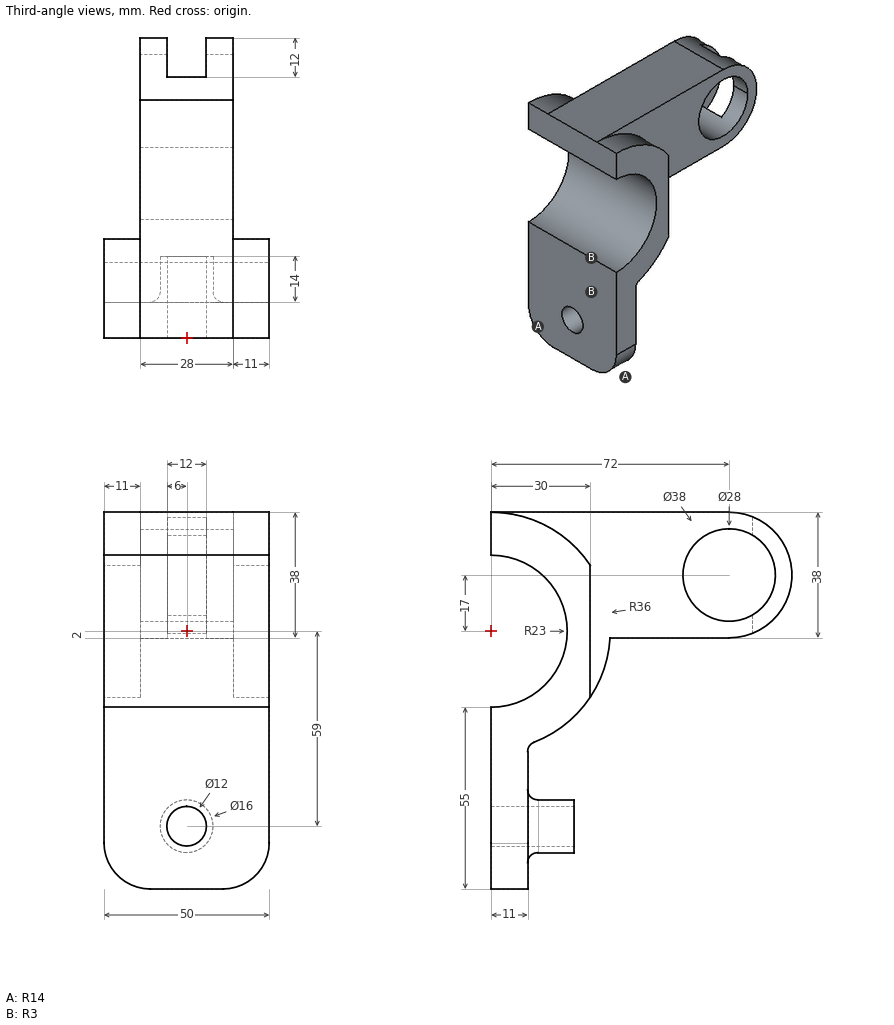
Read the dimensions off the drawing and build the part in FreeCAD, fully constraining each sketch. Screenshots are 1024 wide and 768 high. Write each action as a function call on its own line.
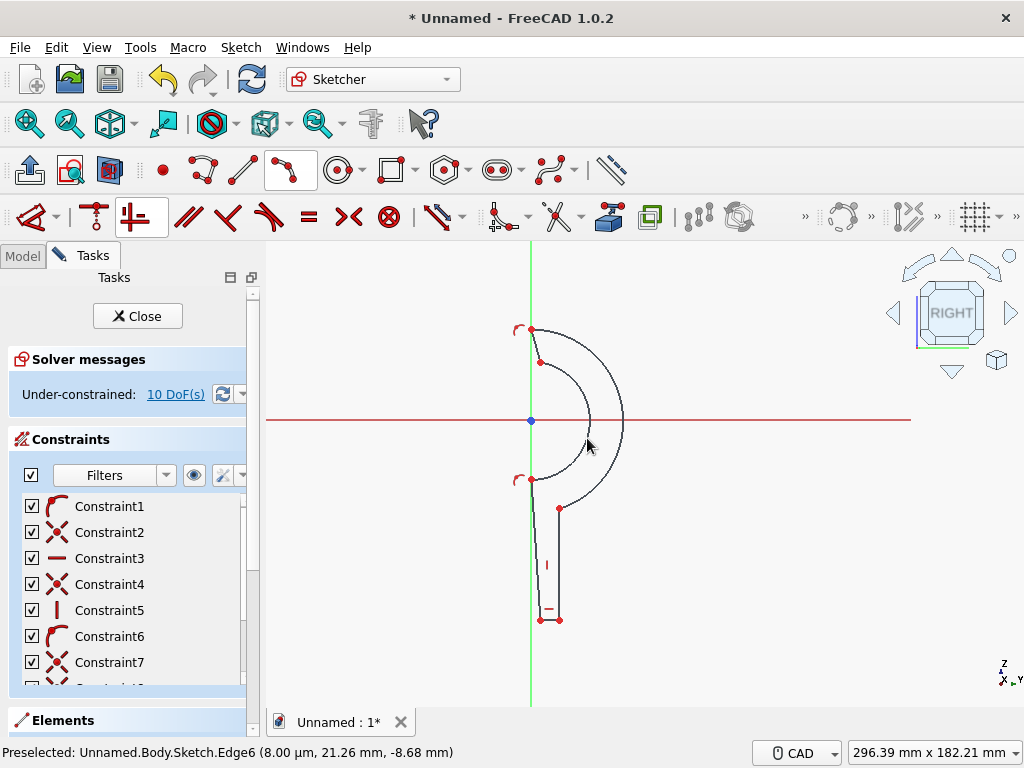
click(534, 522)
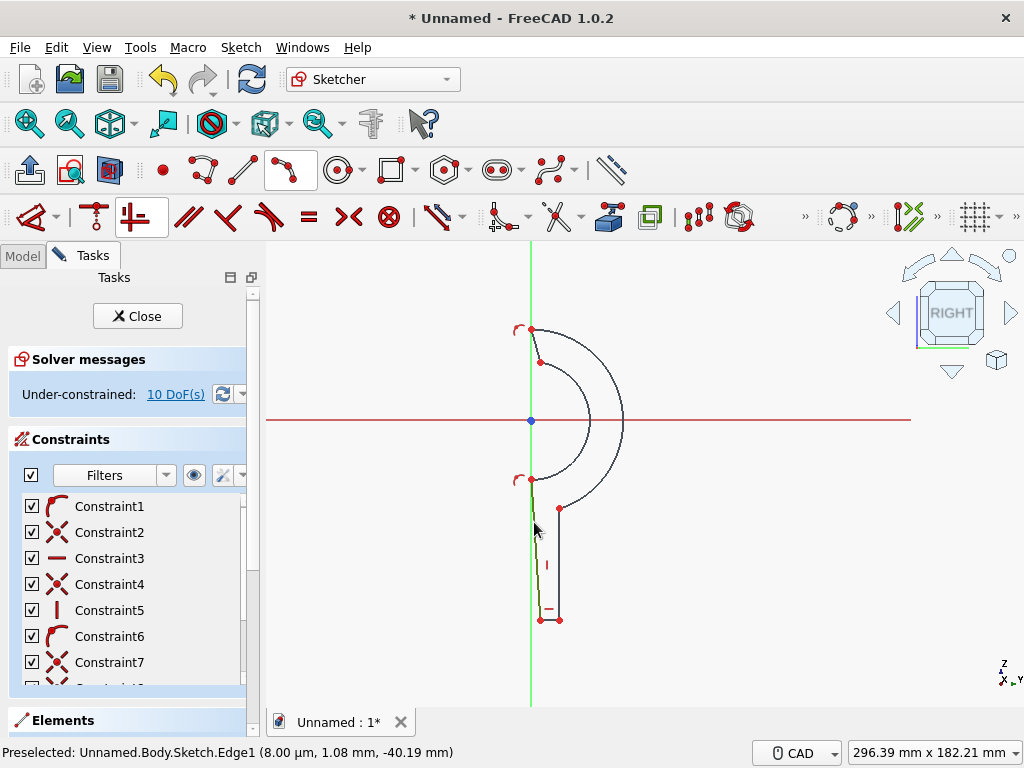
click(162, 218)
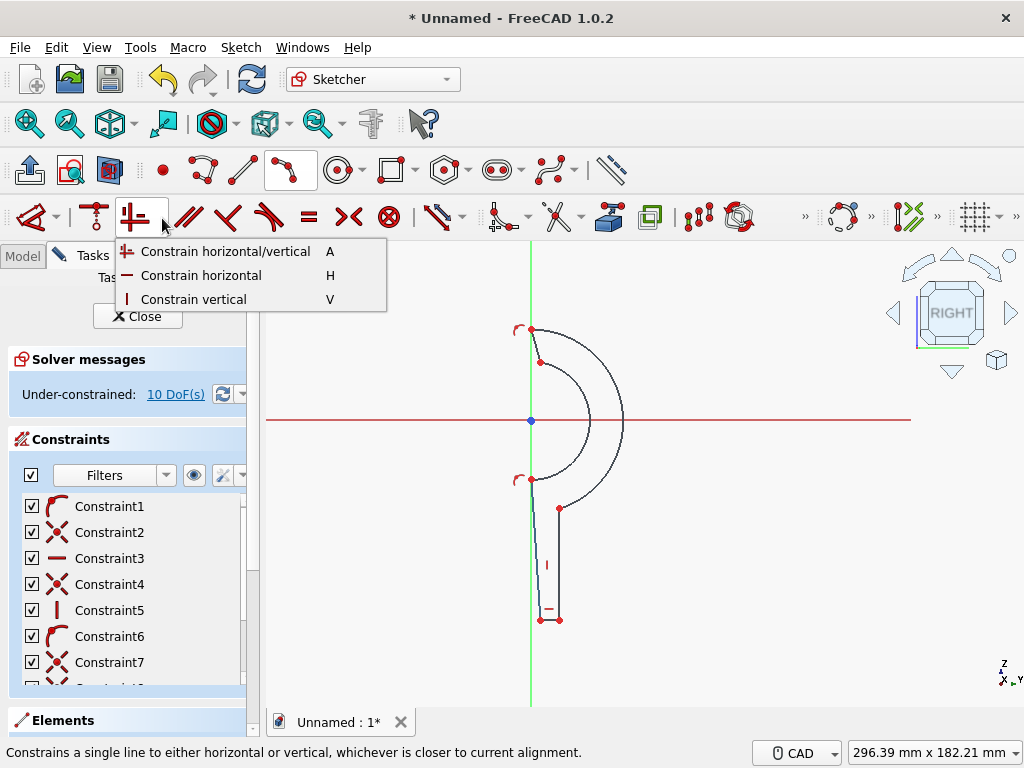
click(251, 299)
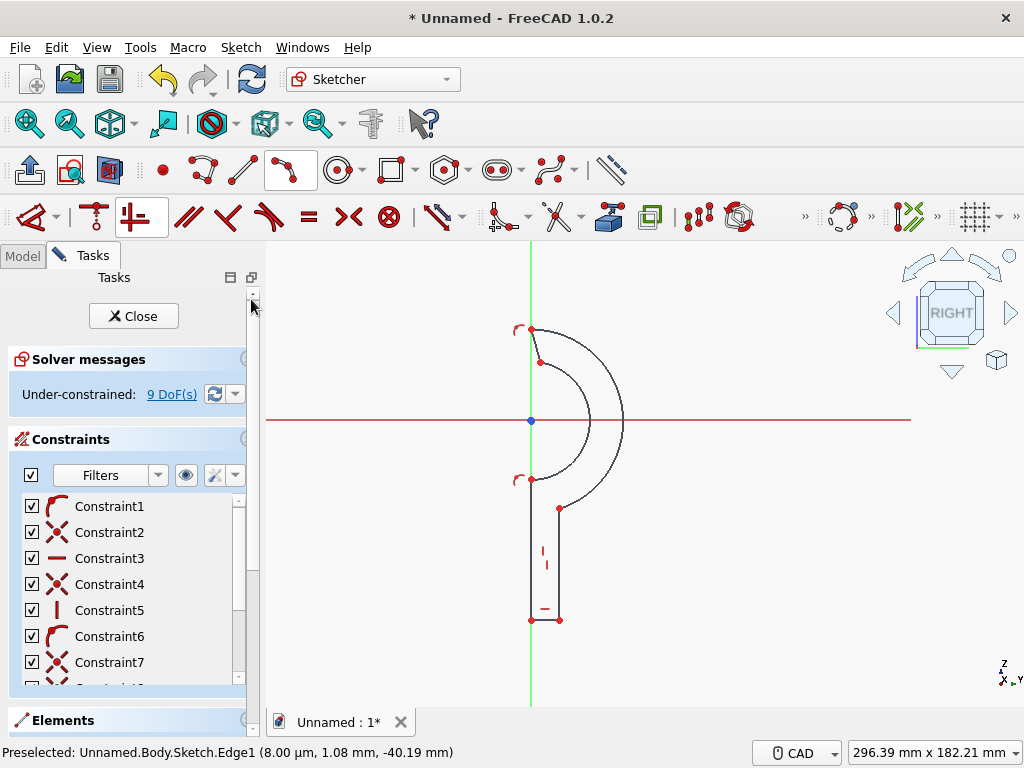
scroll(534, 339, up, 2)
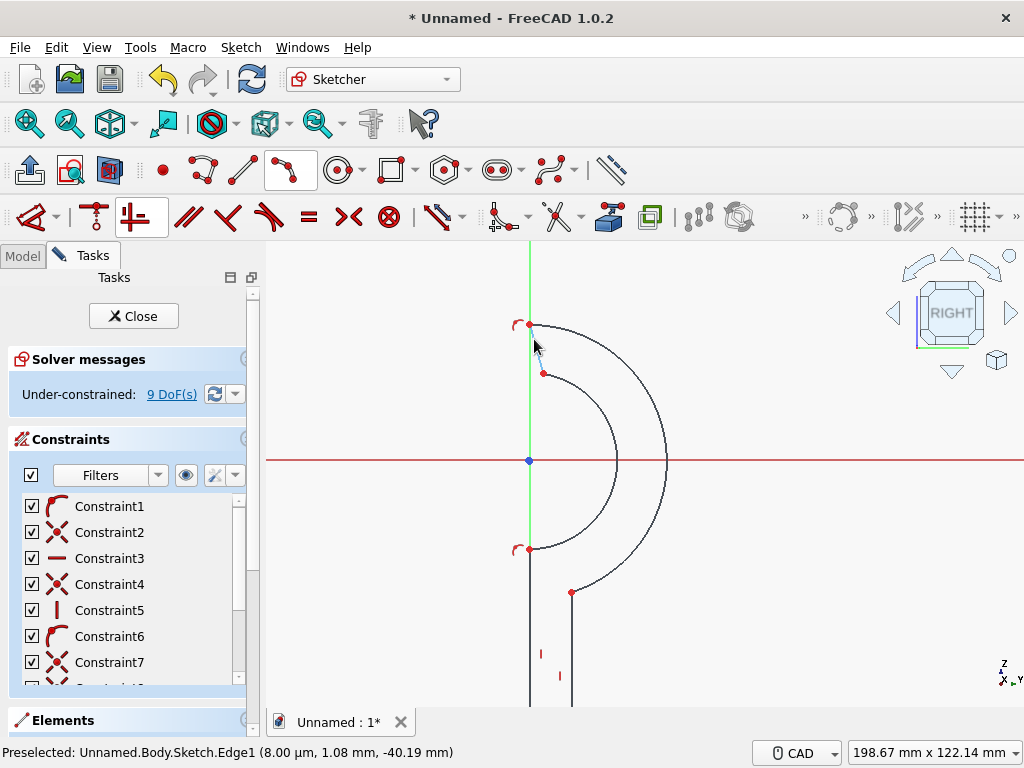
click(534, 340)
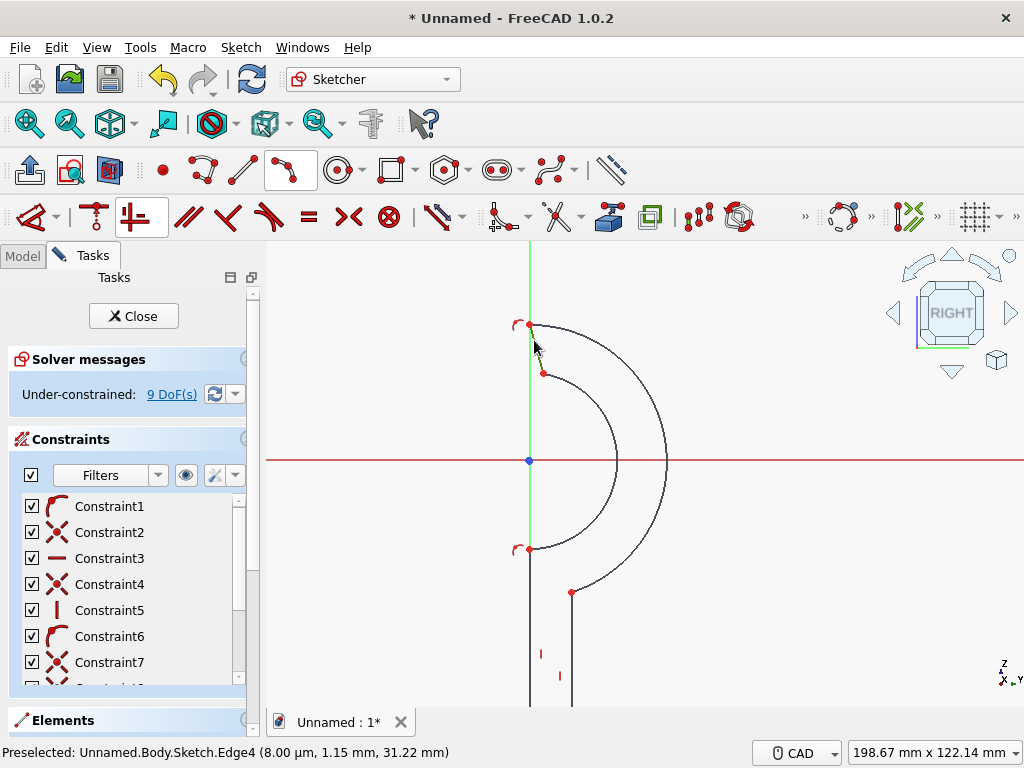
key(v)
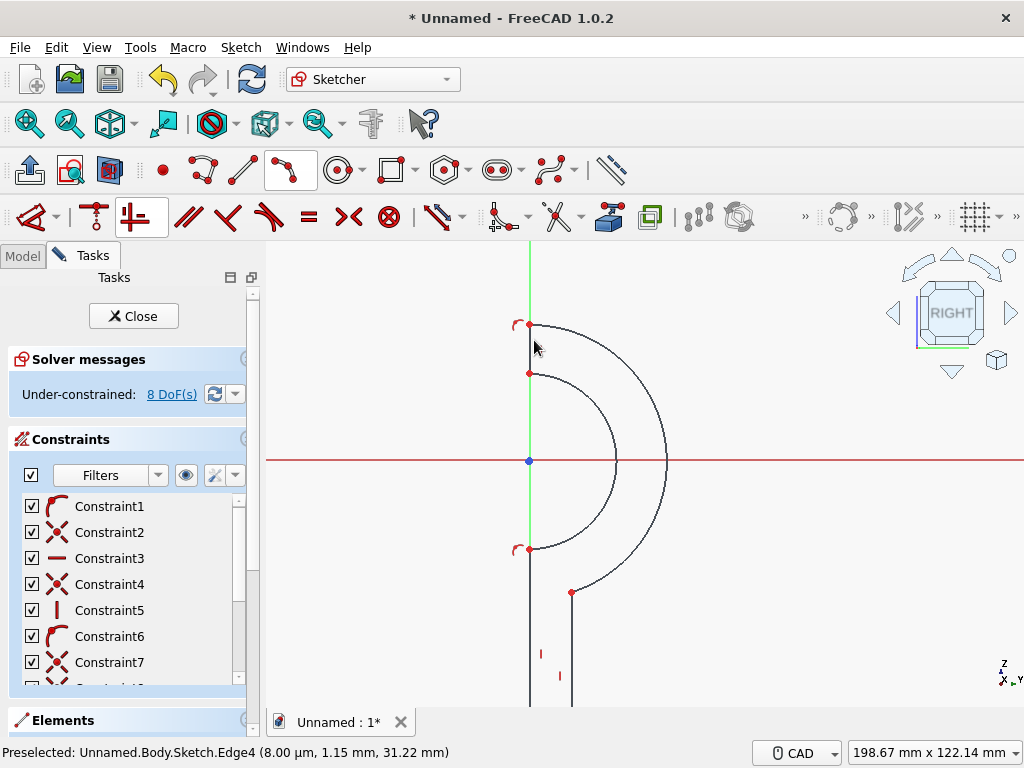
click(655, 517)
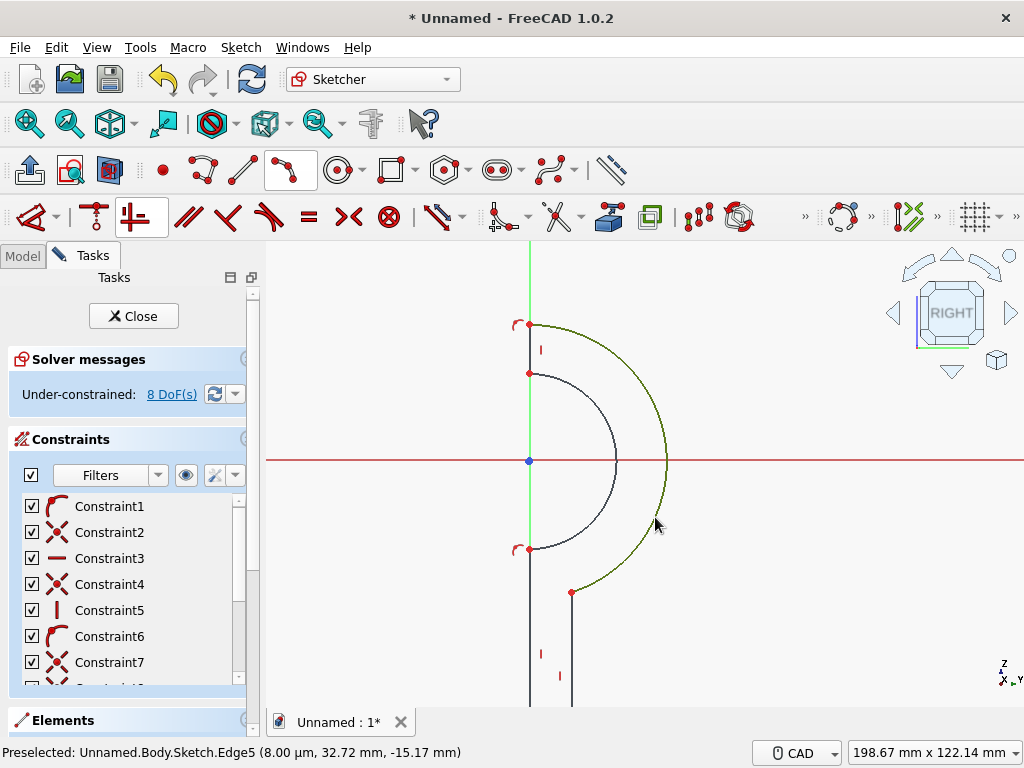
click(600, 513)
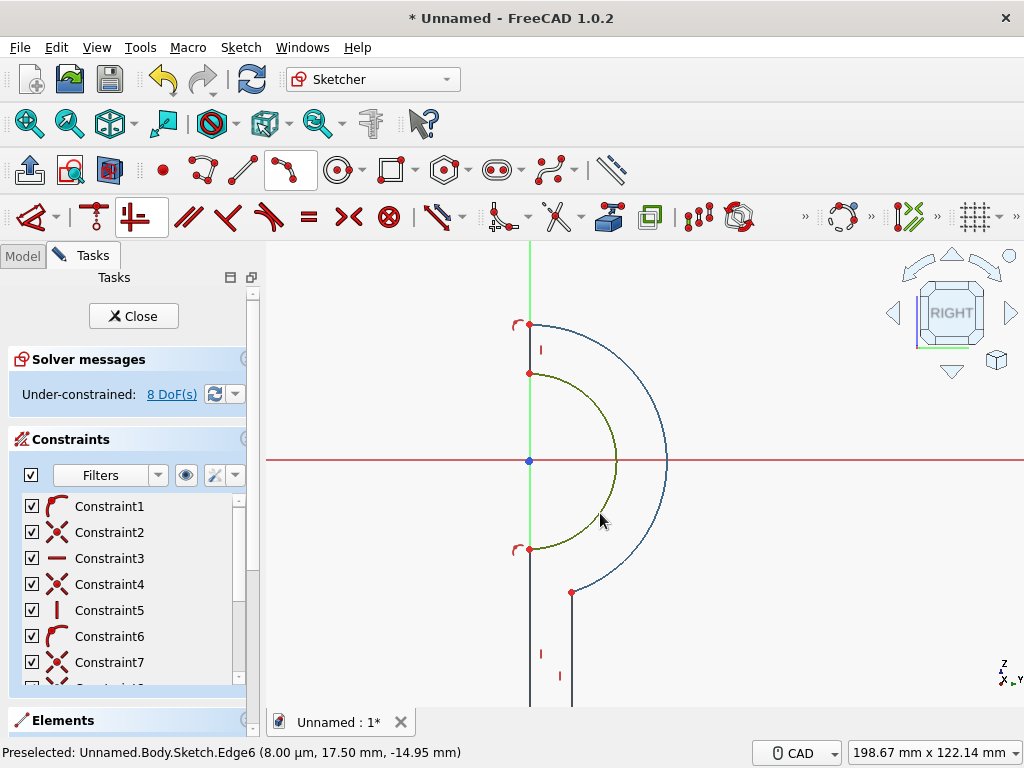
click(94, 218)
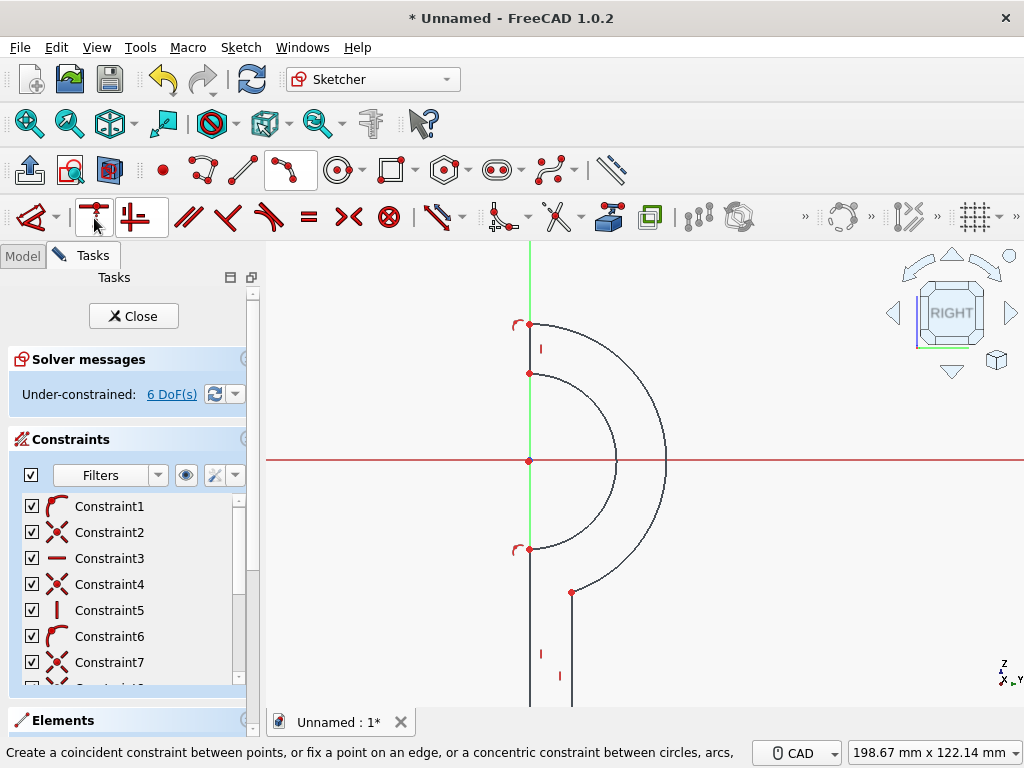
drag(519, 450, 540, 472)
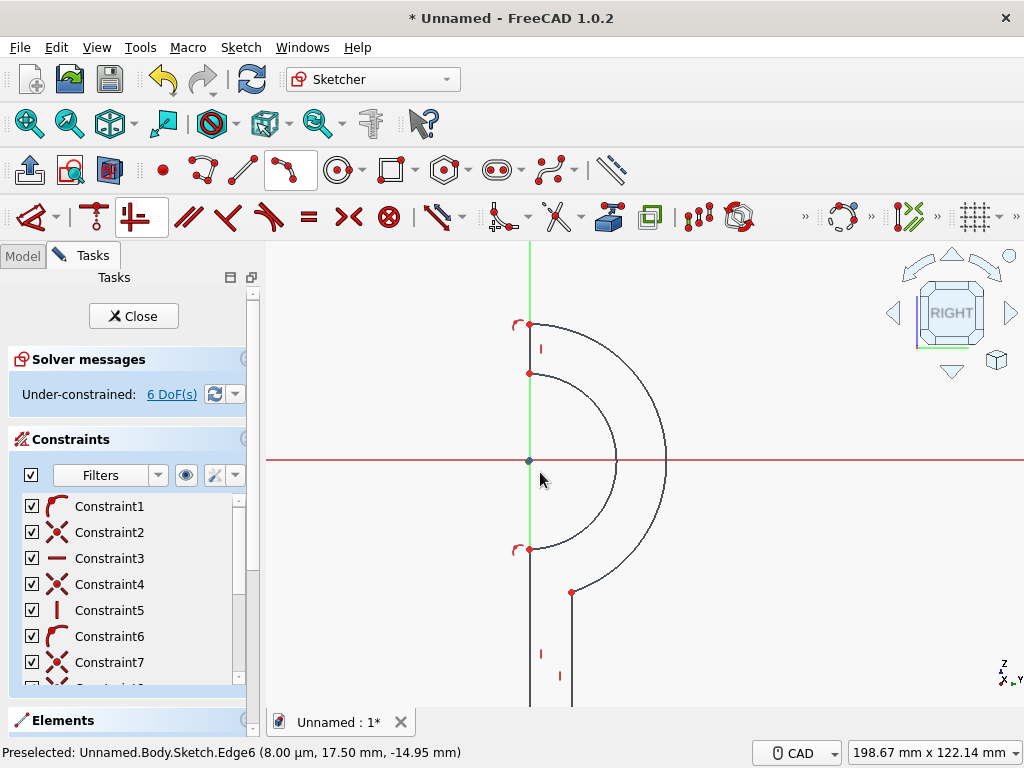
click(94, 218)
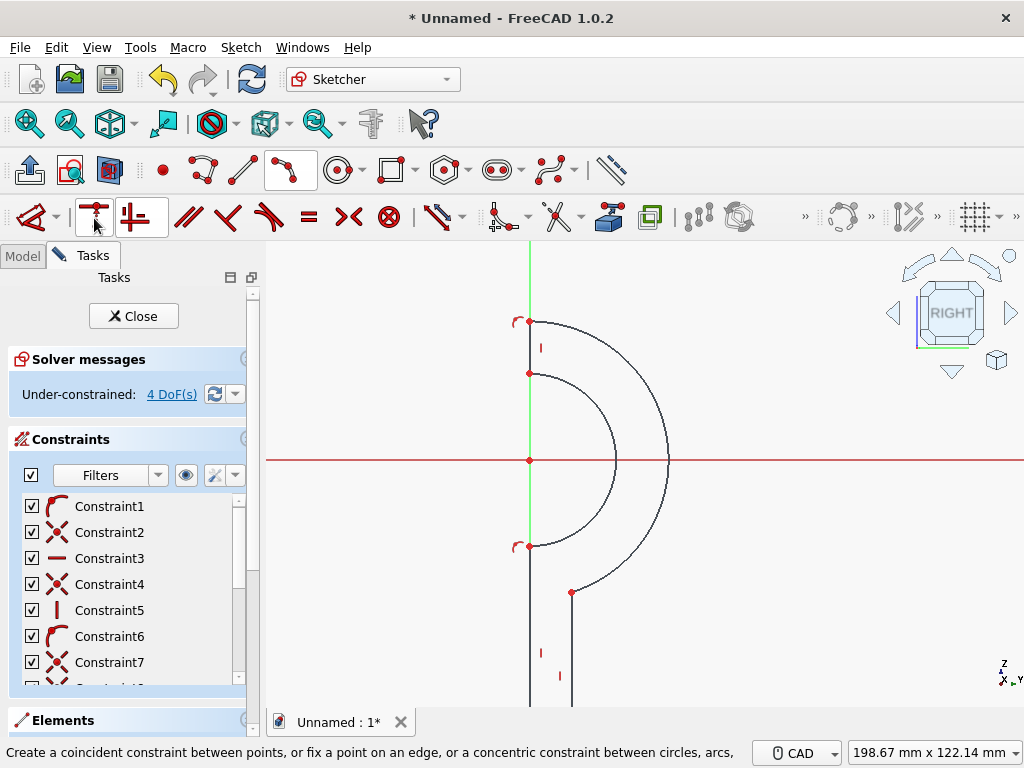
click(32, 218)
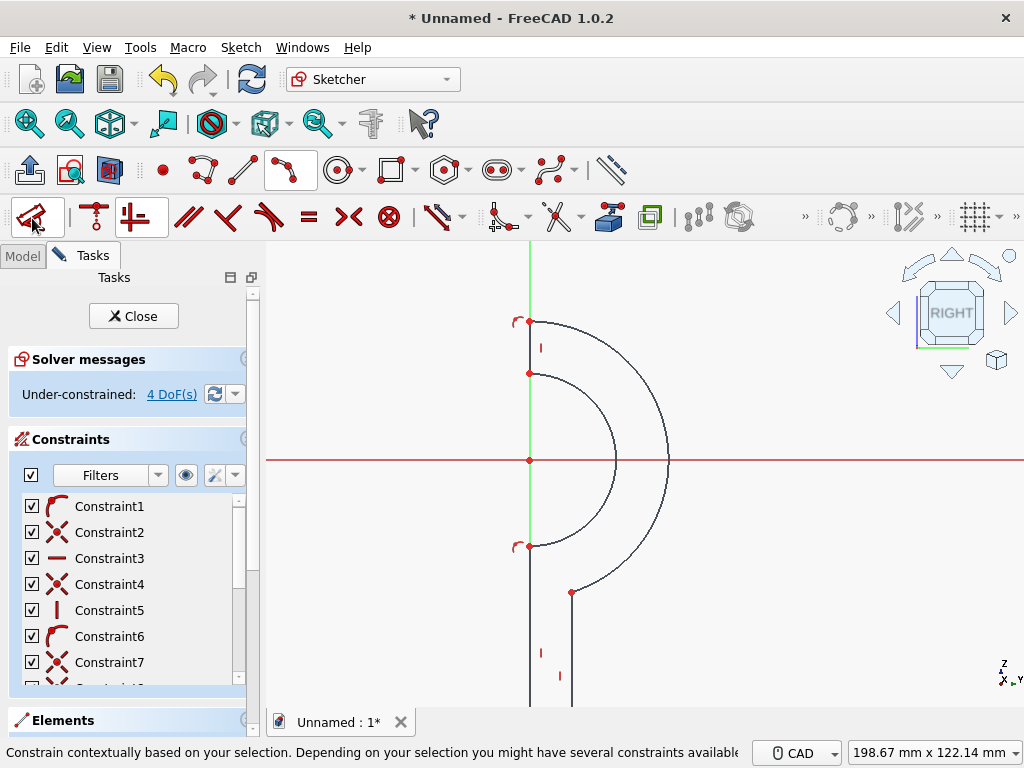
click(657, 516)
click(686, 529)